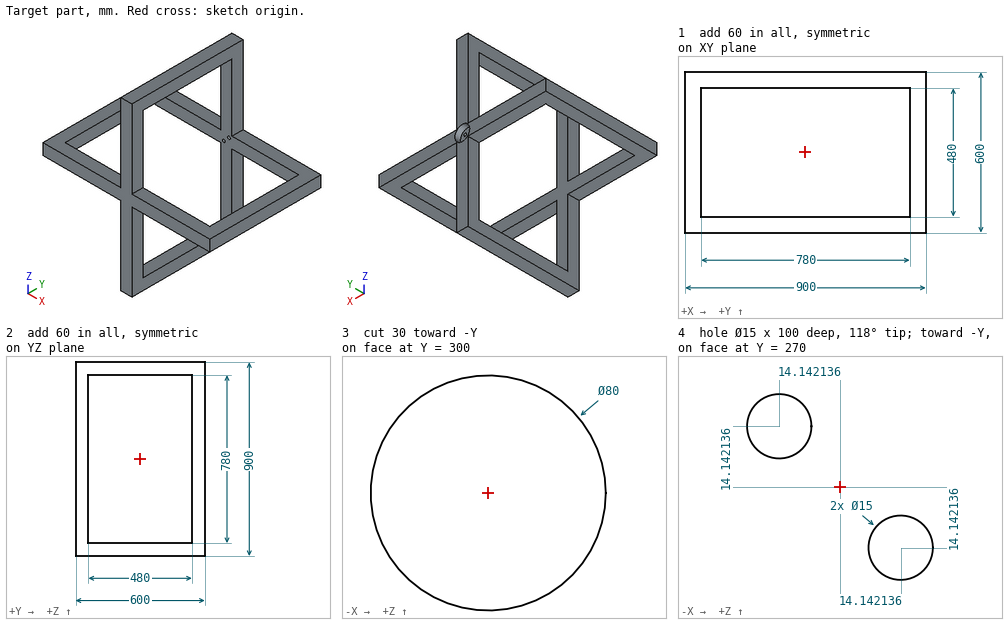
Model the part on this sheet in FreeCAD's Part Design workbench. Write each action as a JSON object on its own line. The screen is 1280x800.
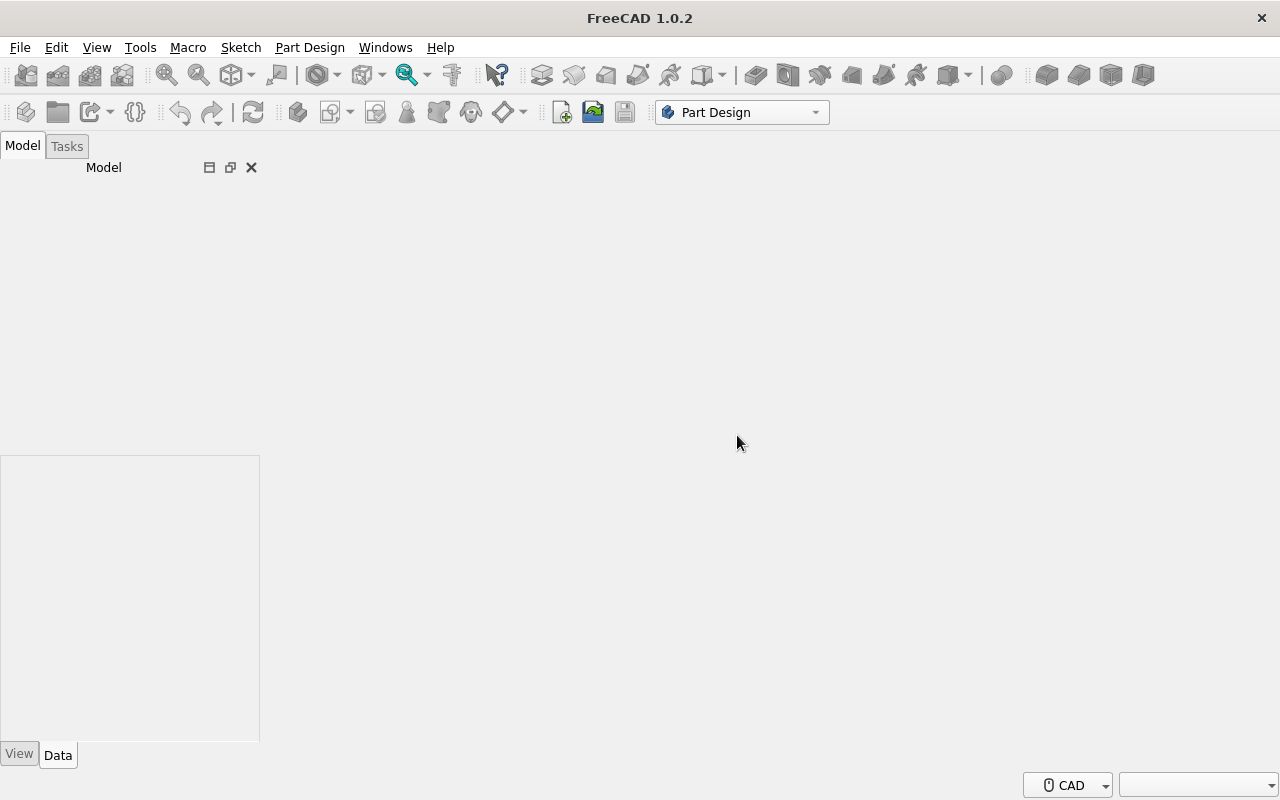
{"action": "left_click", "coordinate": [562, 112]}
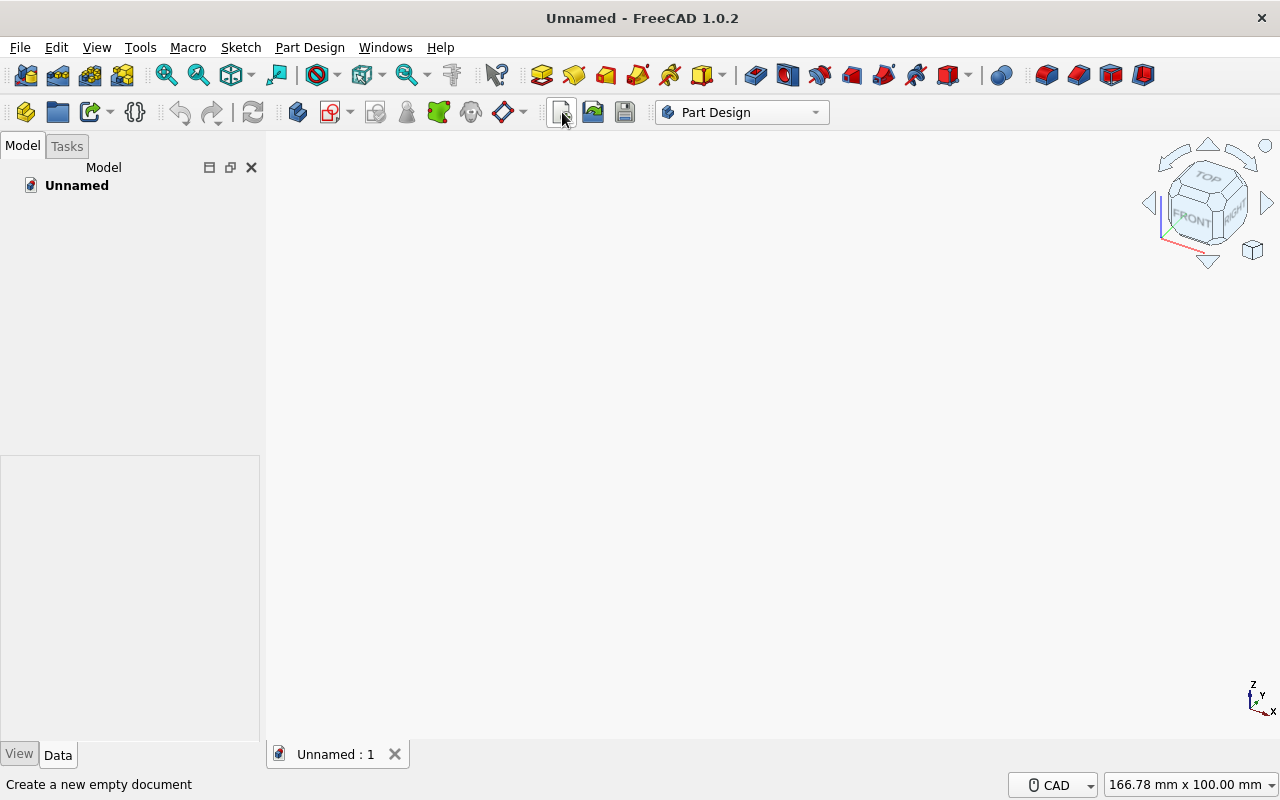
{"action": "left_click", "coordinate": [330, 112]}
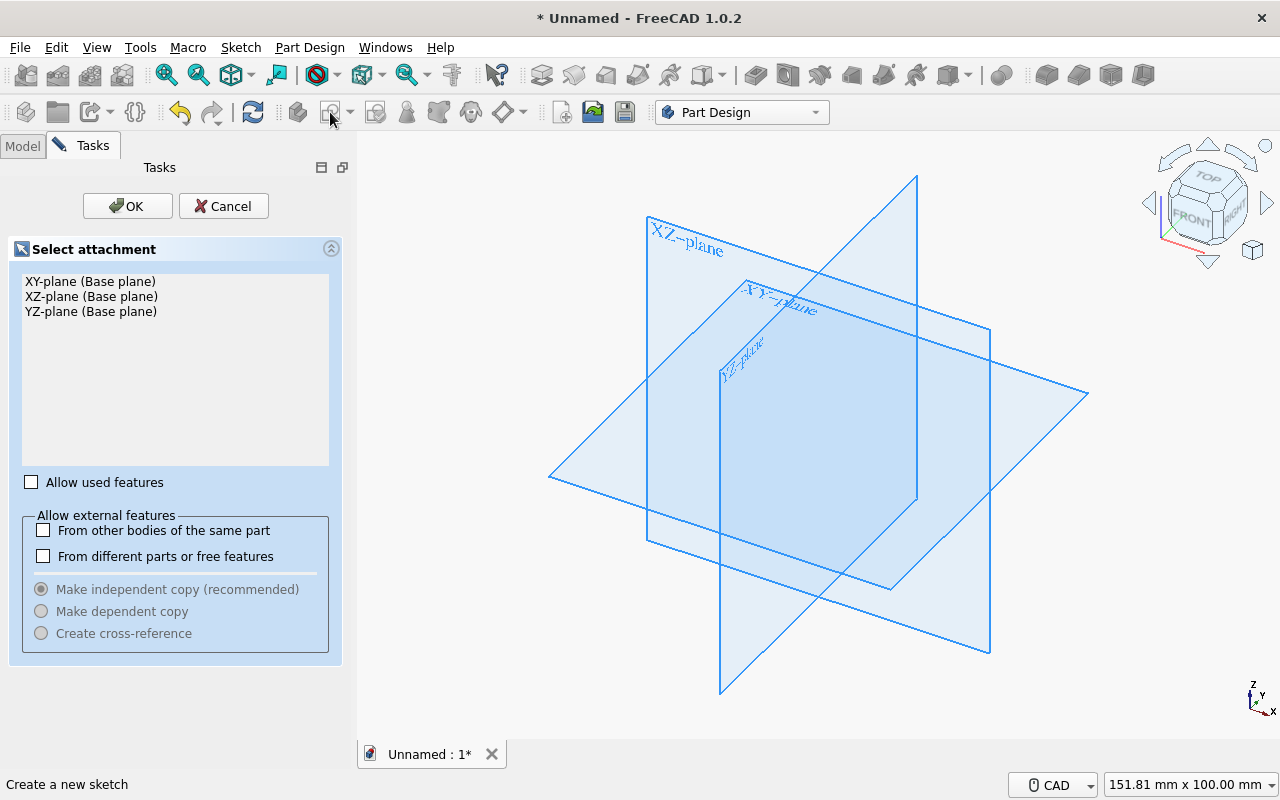
{"action": "left_click", "coordinate": [82, 282]}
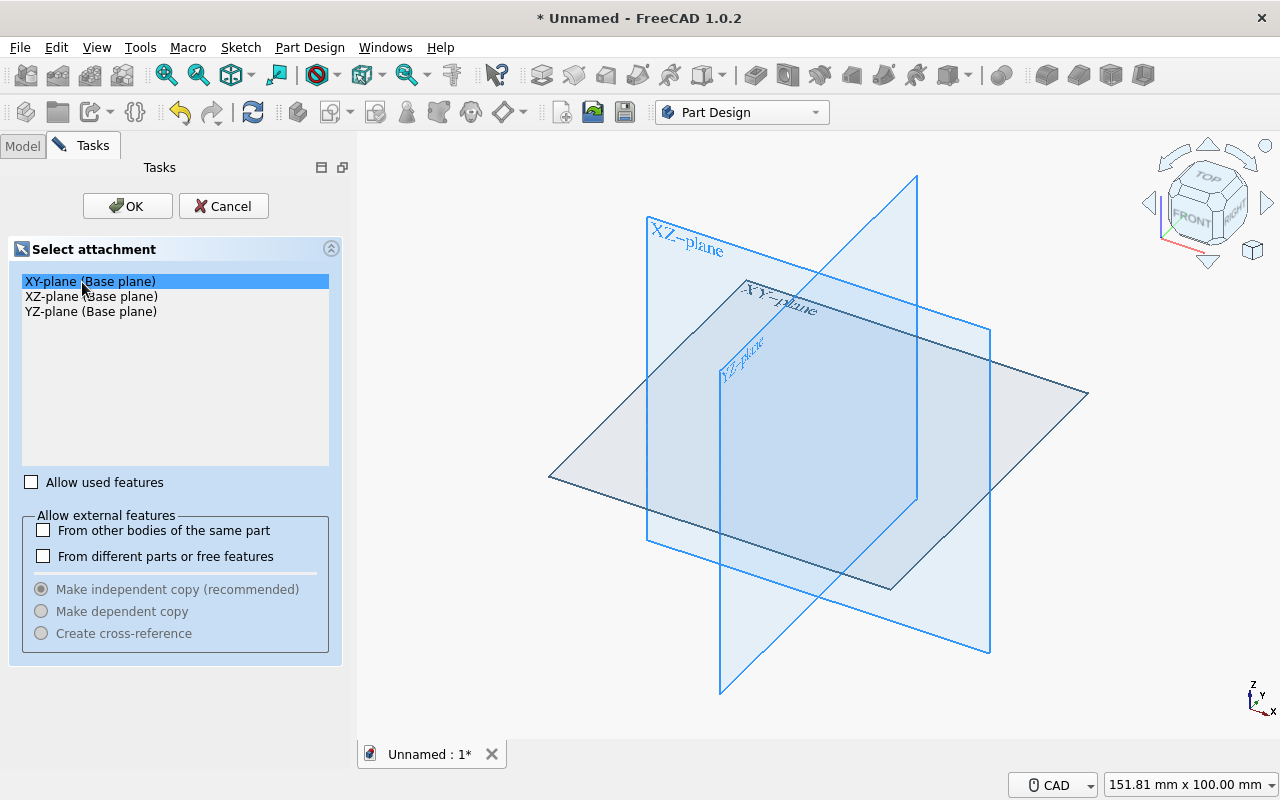
{"action": "left_click", "coordinate": [128, 206]}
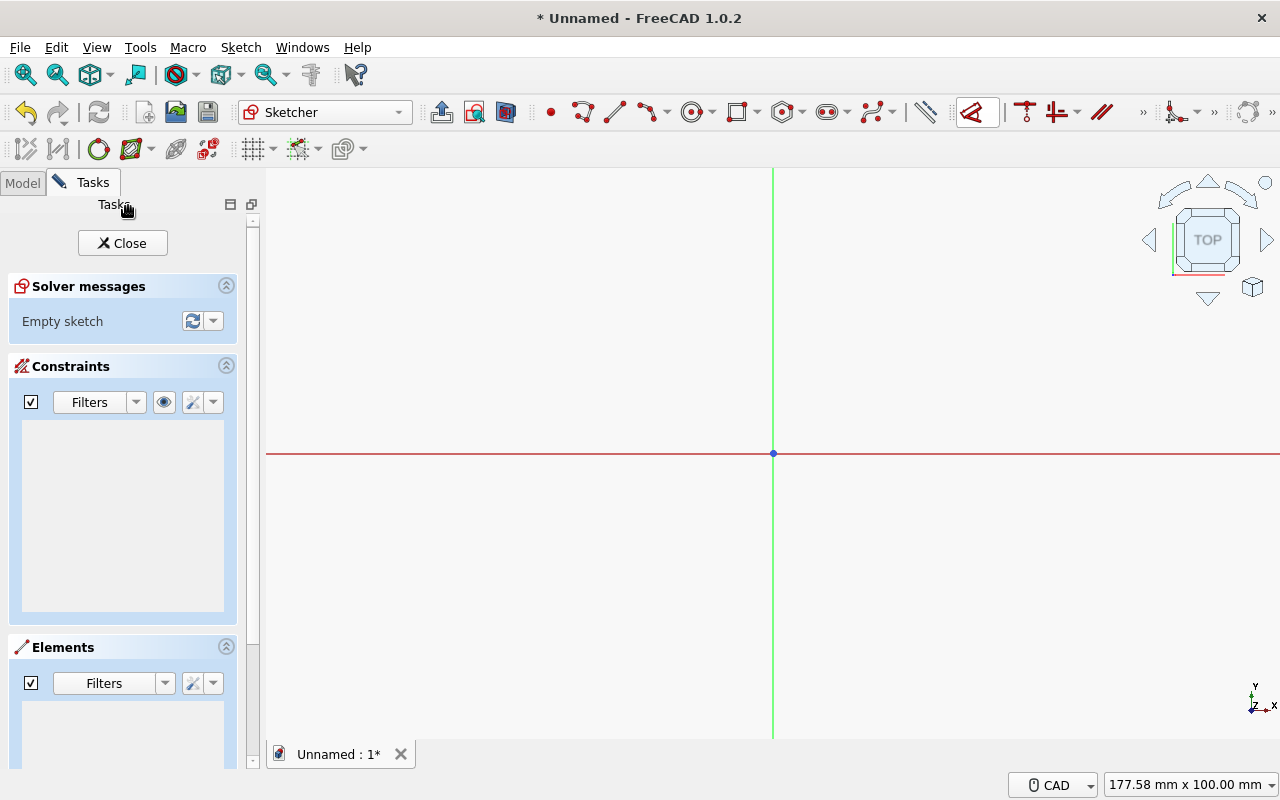
{"action": "scroll", "coordinate": [696, 454], "scroll_direction": "down", "scroll_amount": 11}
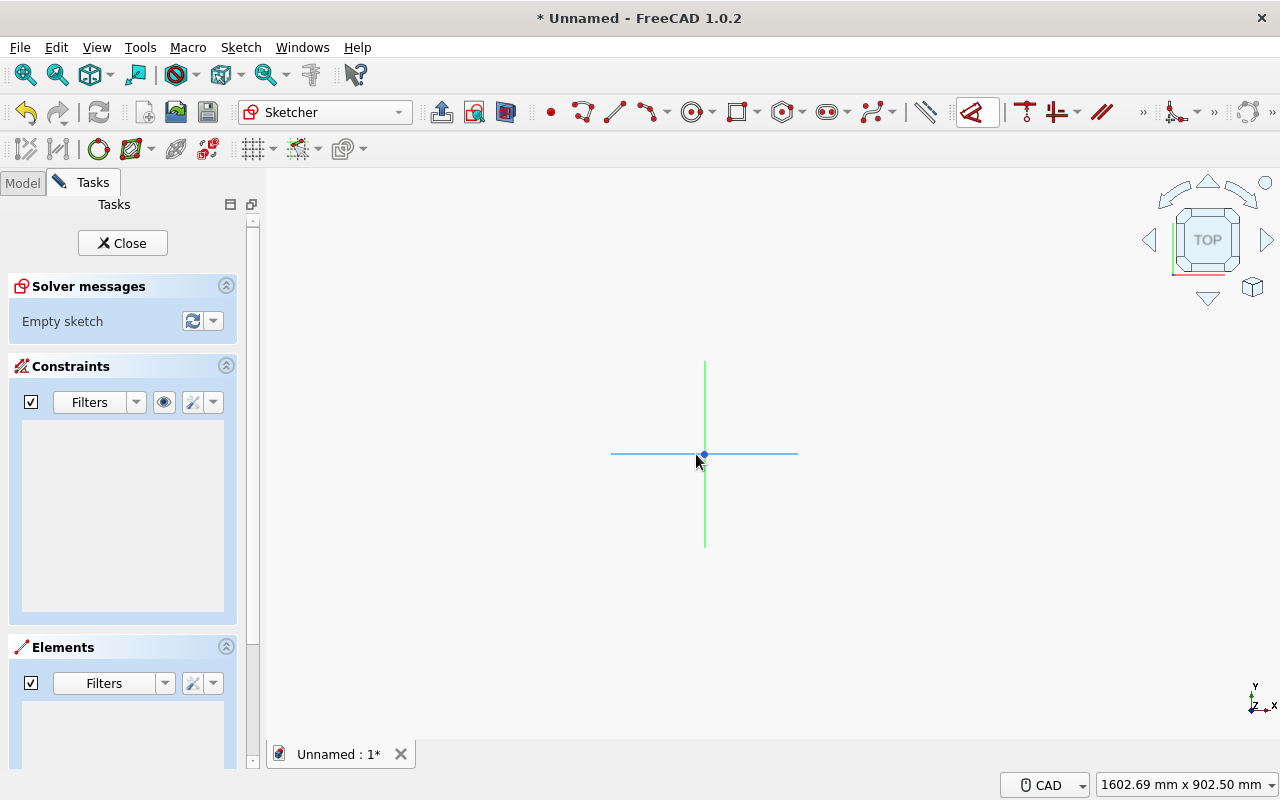
{"action": "left_click", "coordinate": [760, 112]}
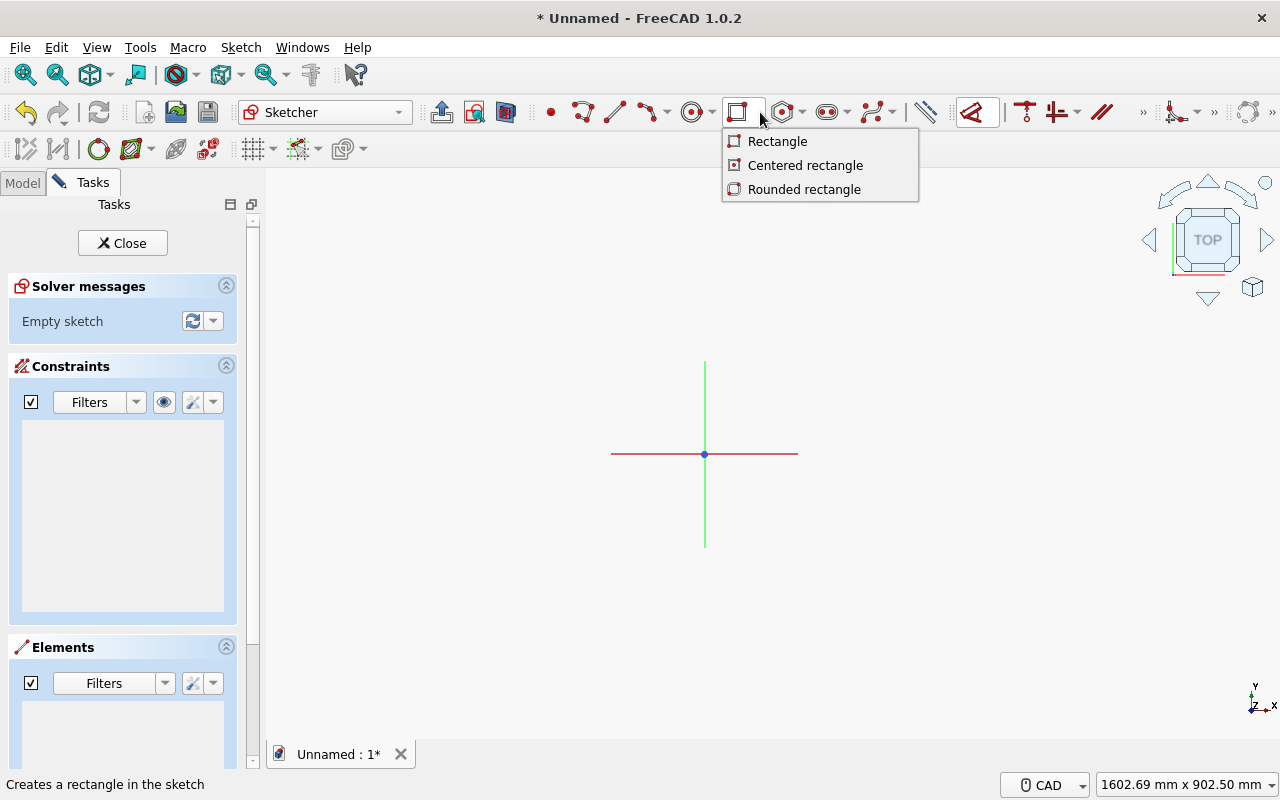
{"action": "left_click", "coordinate": [820, 165]}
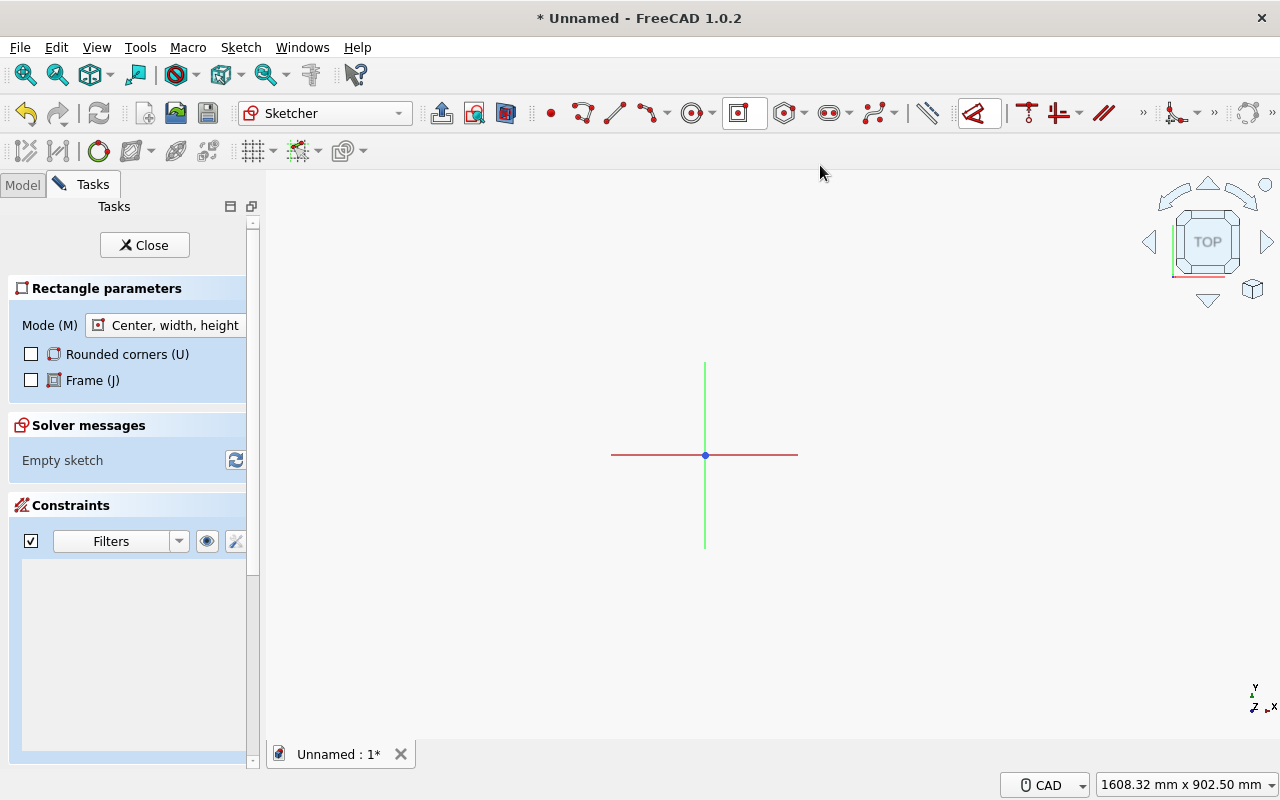
{"action": "left_click", "coordinate": [705, 455]}
{"action": "mouse_move", "coordinate": [989, 266]}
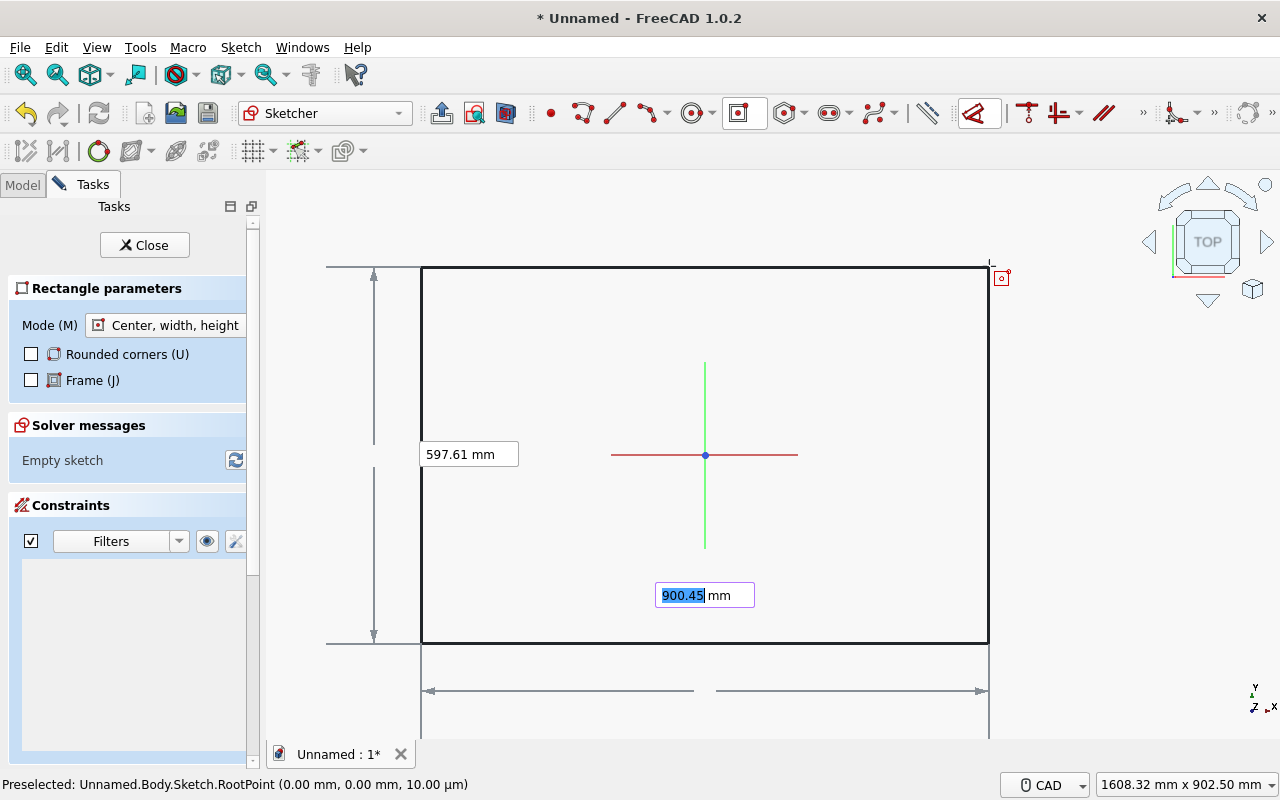
{"action": "type", "text": "900"}
{"action": "key", "text": "Tab"}
{"action": "type", "text": "600"}
{"action": "key", "text": "Return"}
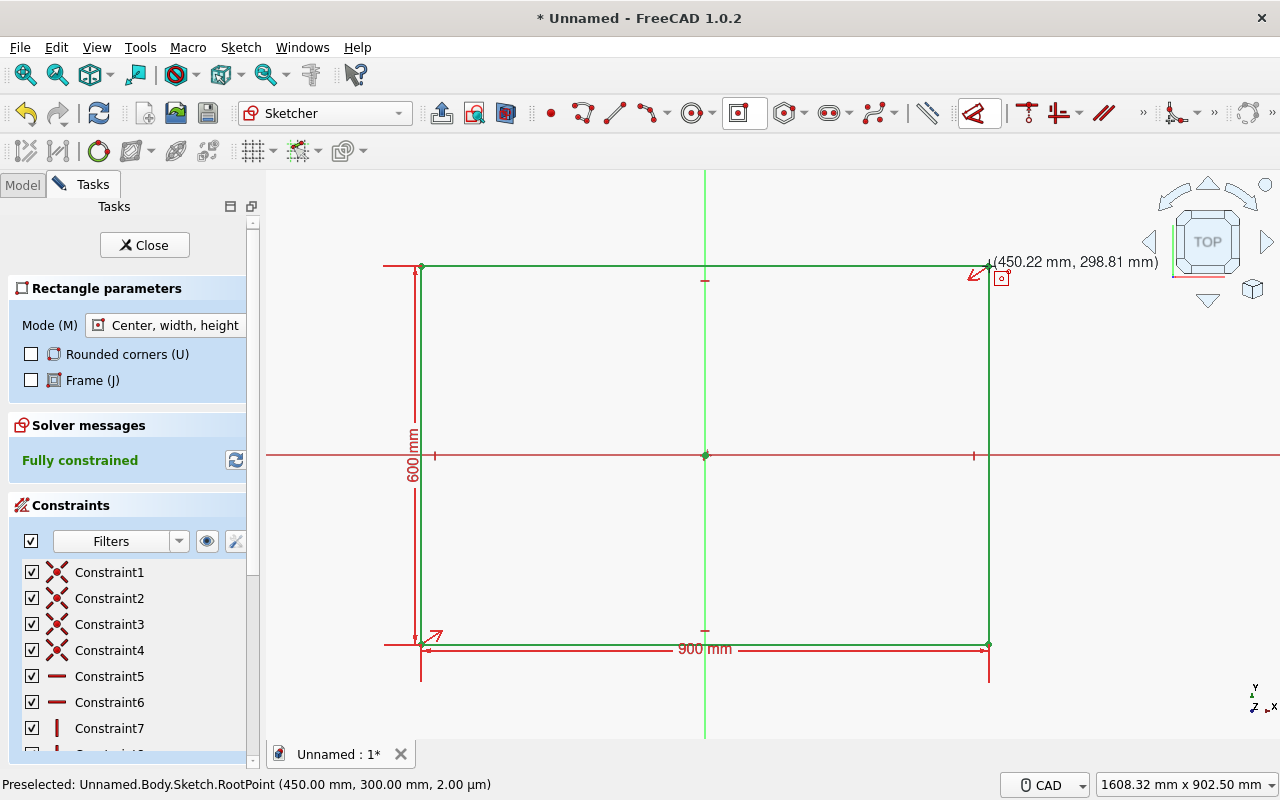
{"action": "left_click", "coordinate": [705, 455]}
{"action": "mouse_move", "coordinate": [951, 304]}